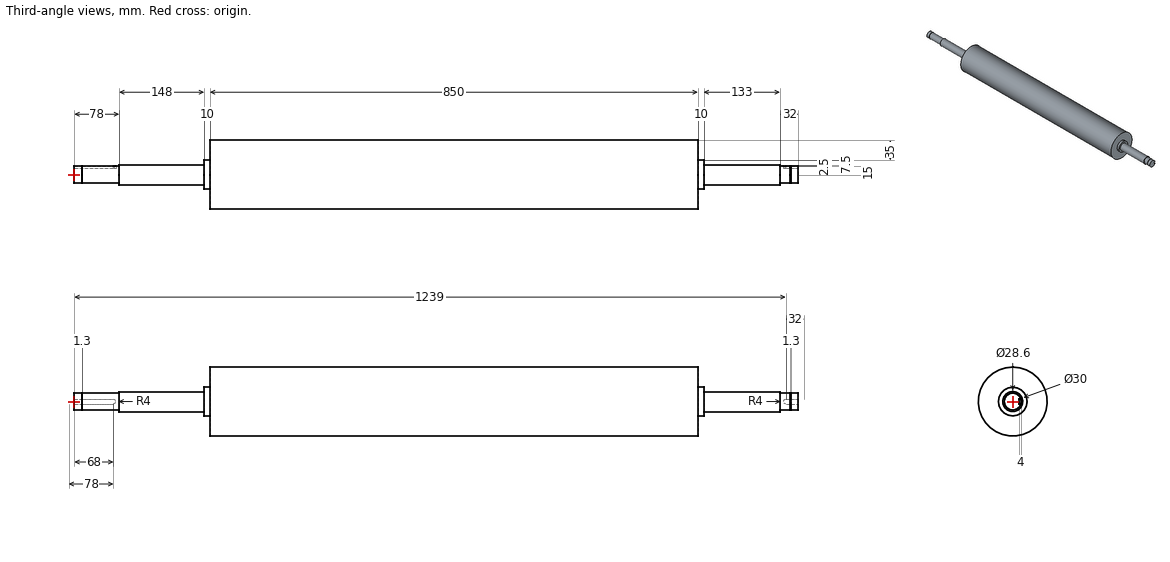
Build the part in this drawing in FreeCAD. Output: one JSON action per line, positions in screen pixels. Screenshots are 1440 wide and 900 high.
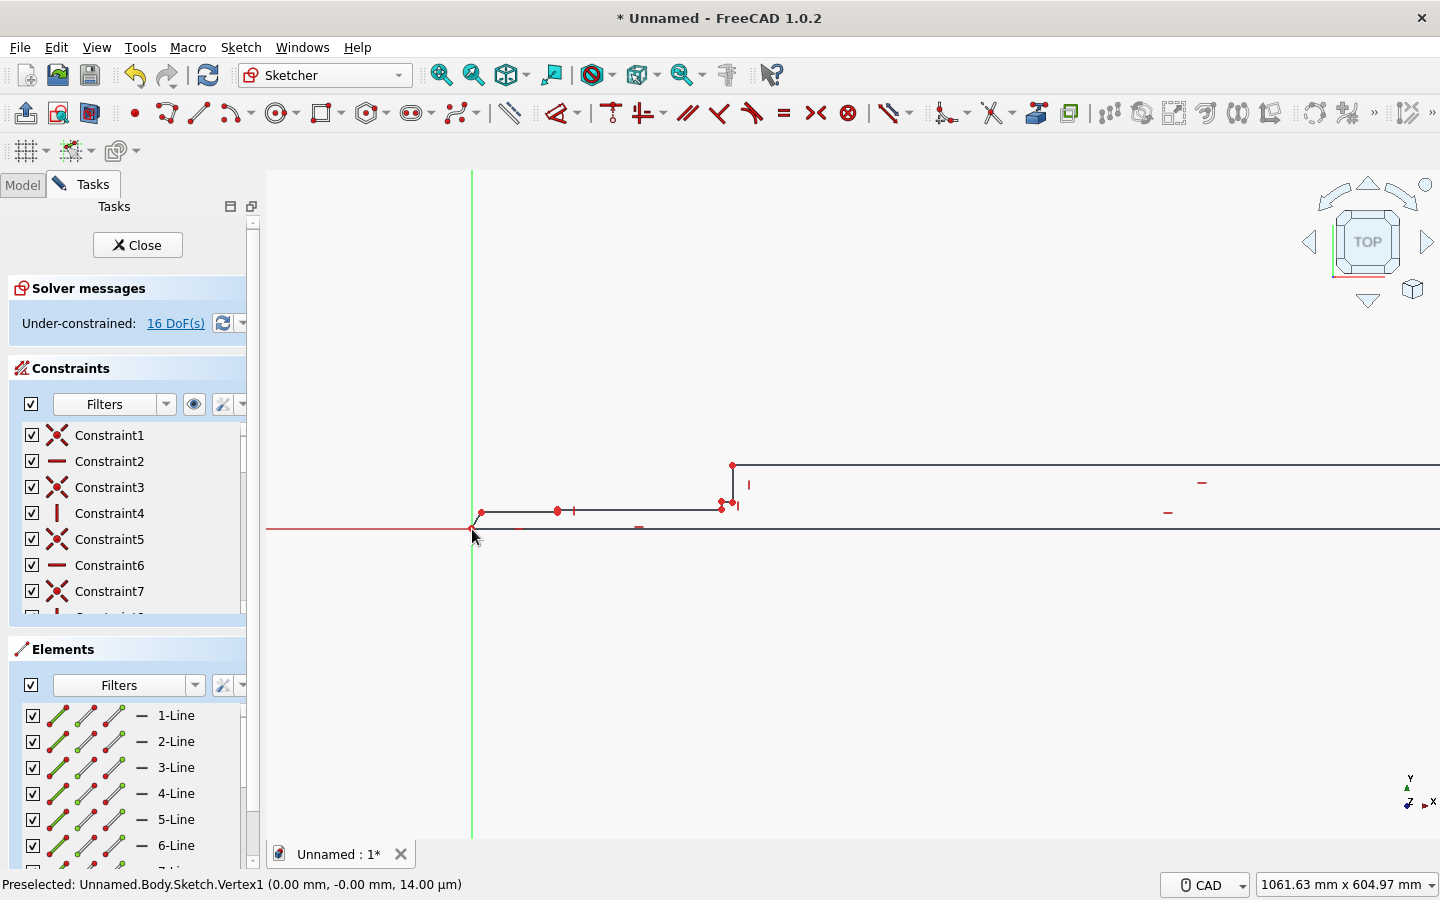
{"action": "scroll", "coordinate": [727, 502], "scroll_direction": "up", "scroll_amount": 5}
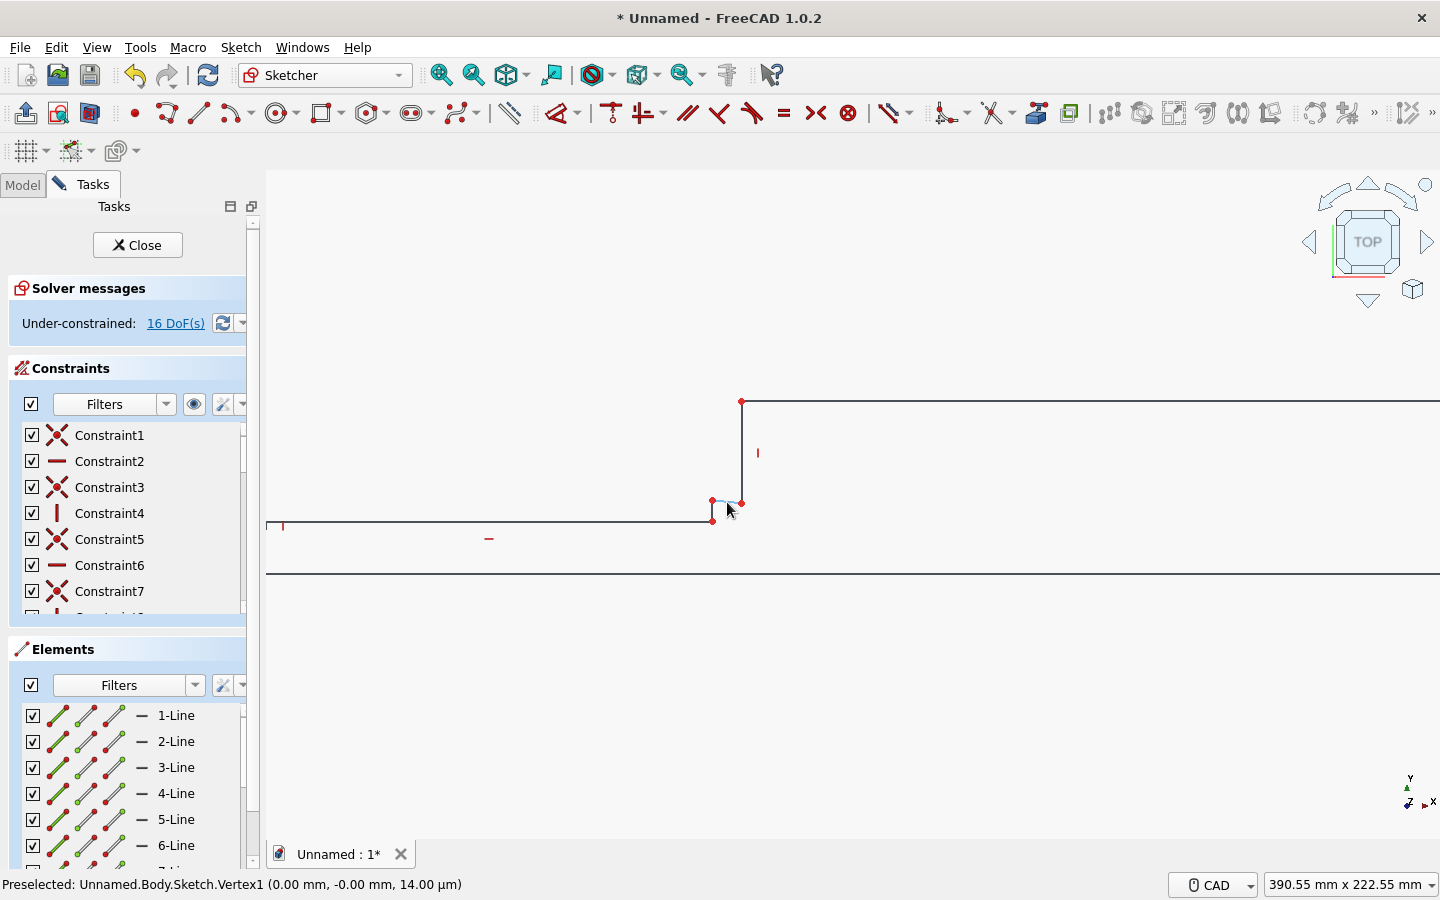
{"action": "left_click", "coordinate": [727, 502]}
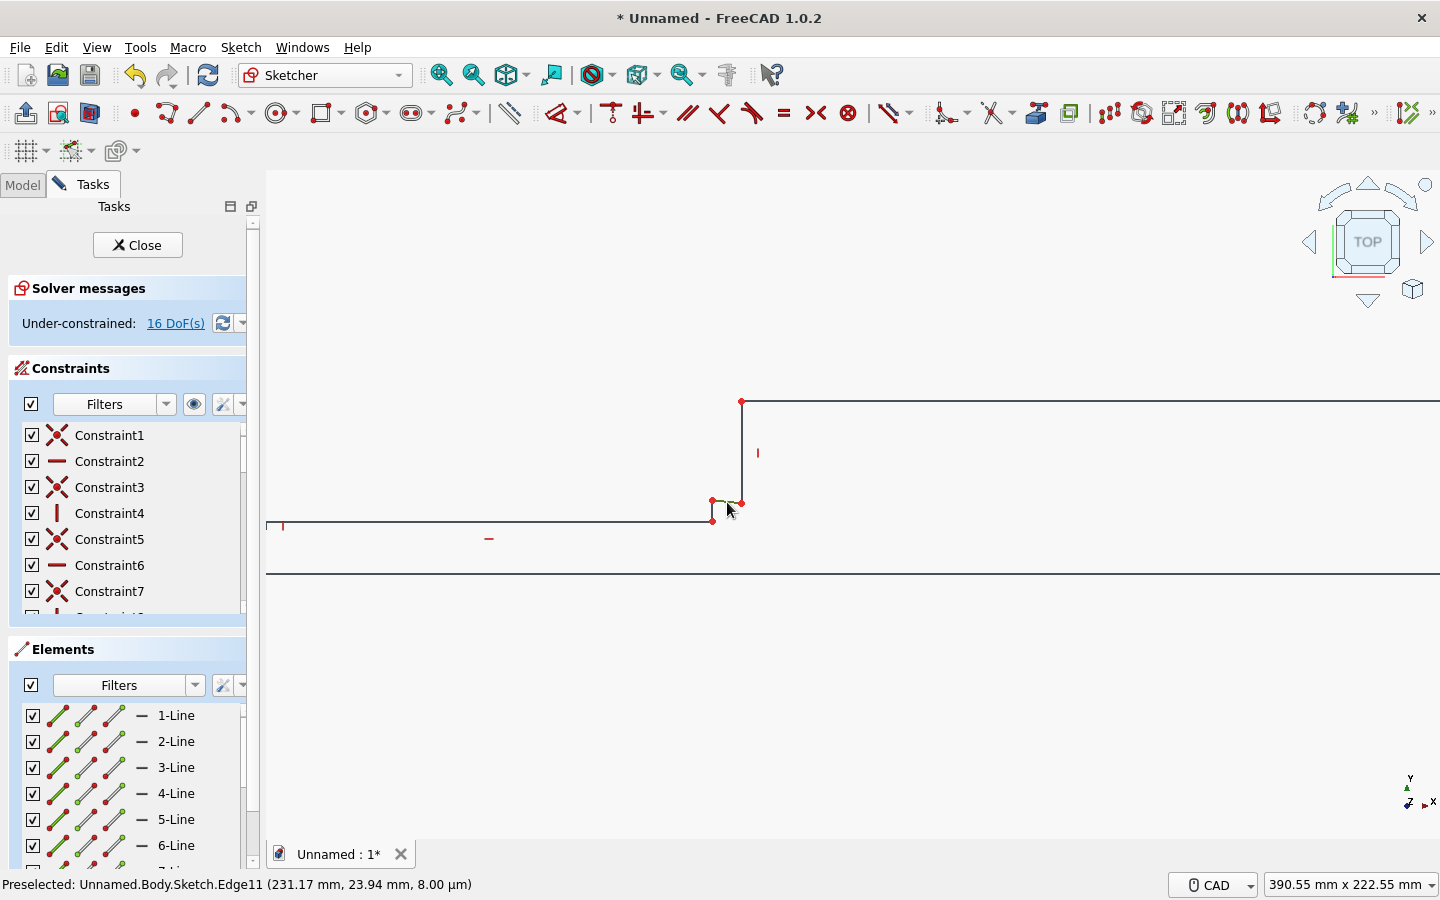
{"action": "left_click", "coordinate": [666, 114]}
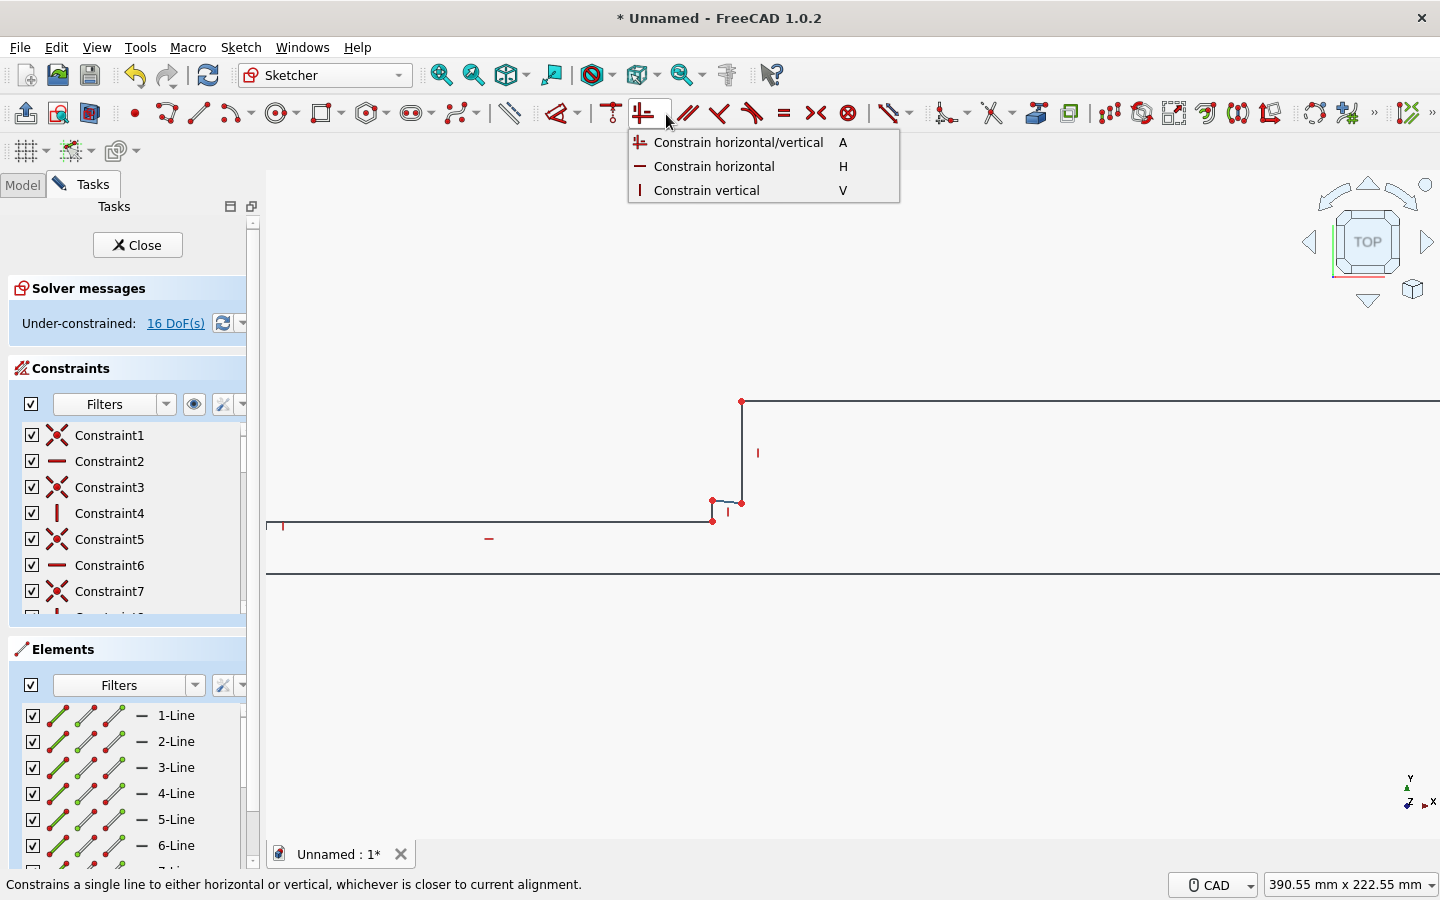
{"action": "left_click", "coordinate": [764, 166]}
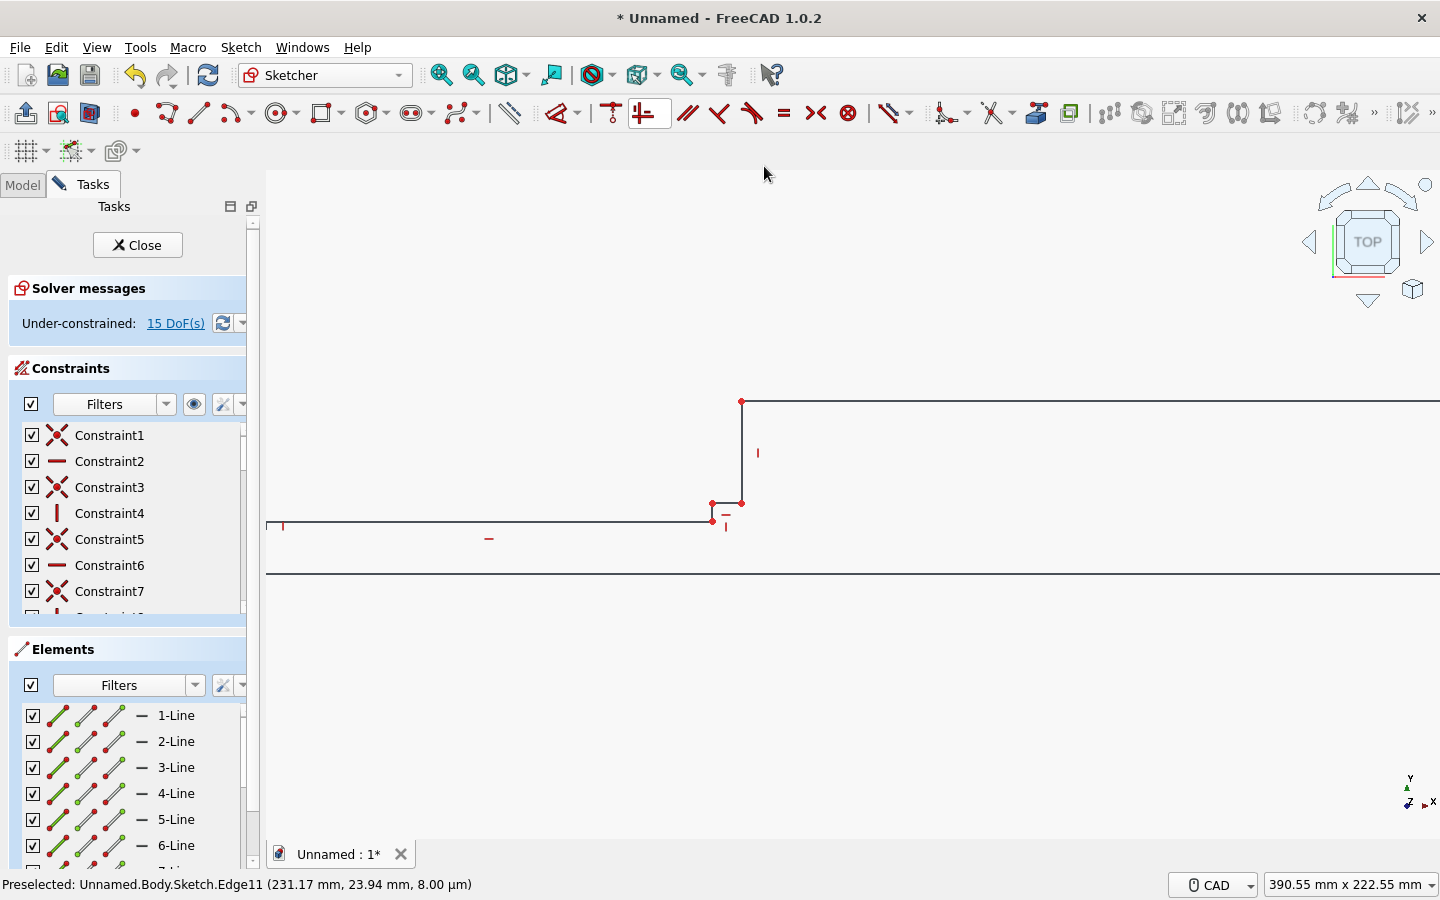
{"action": "scroll", "coordinate": [558, 509], "scroll_direction": "down", "scroll_amount": 9}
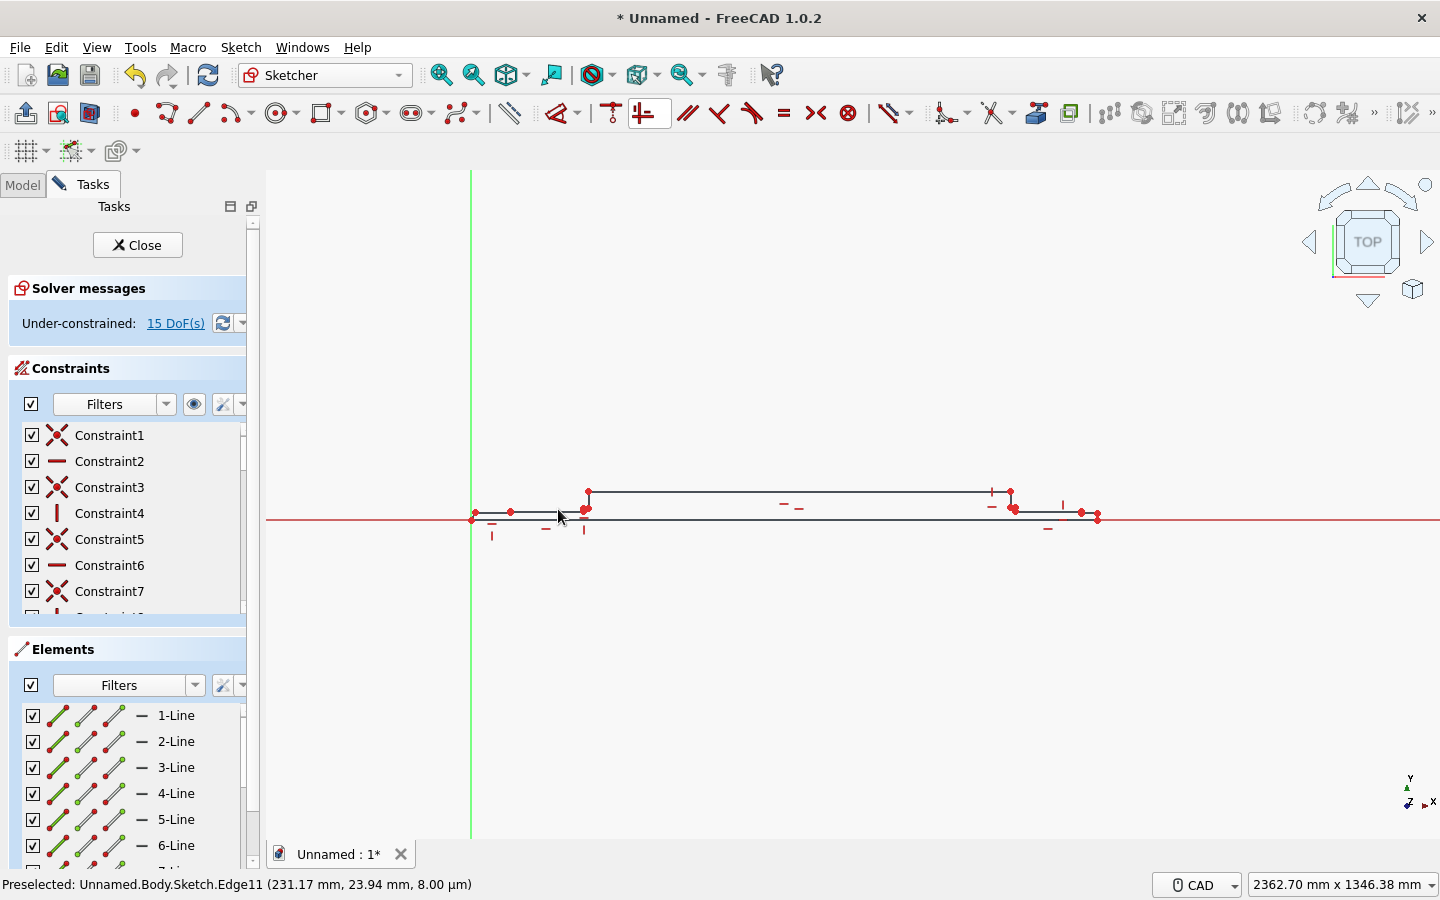
{"action": "scroll", "coordinate": [474, 515], "scroll_direction": "up", "scroll_amount": 9}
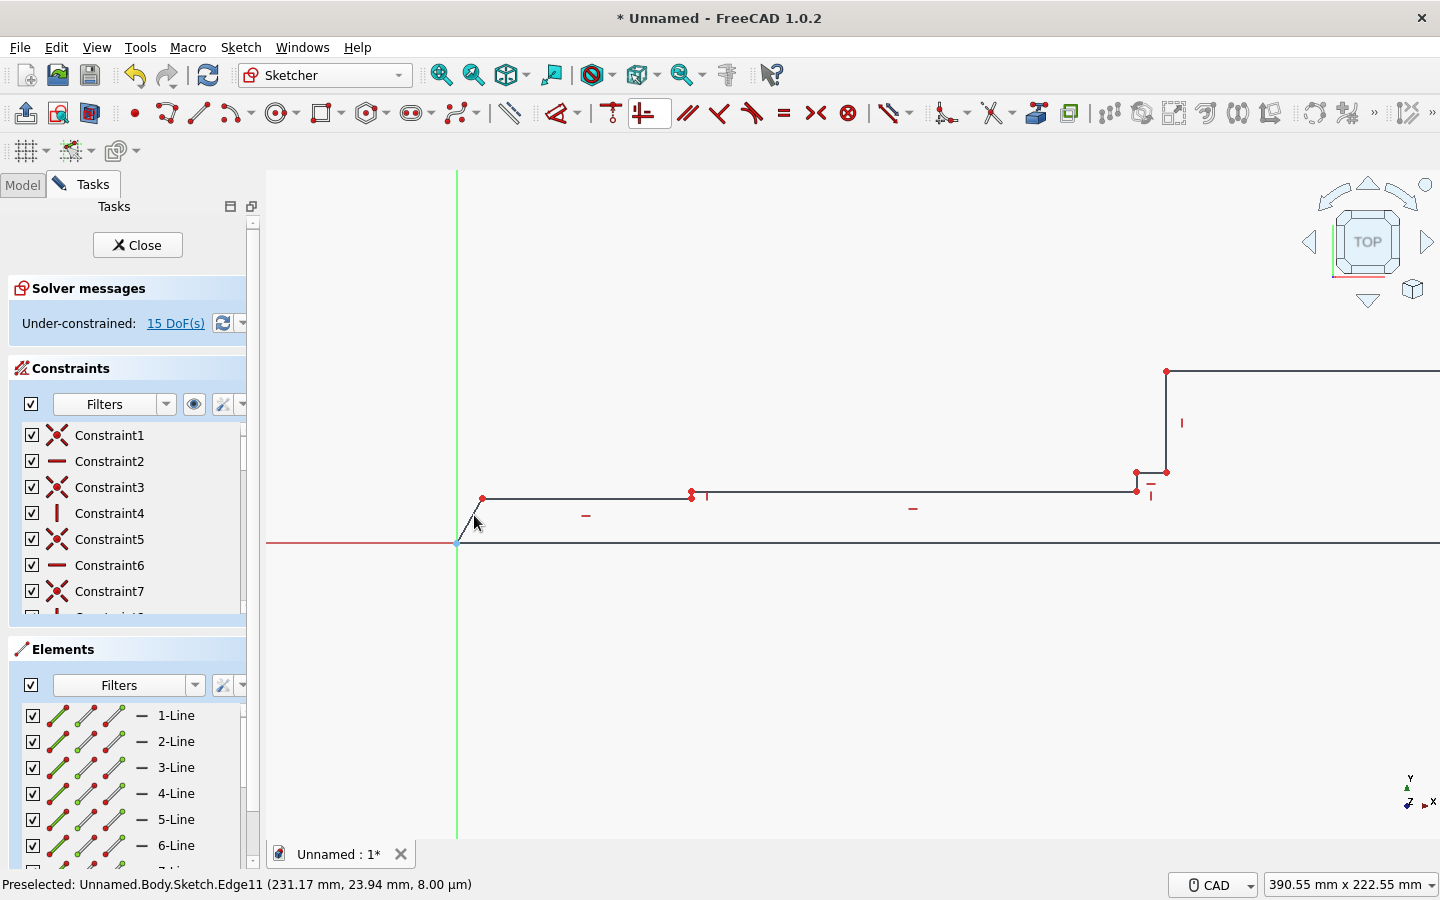
{"action": "left_click", "coordinate": [475, 512]}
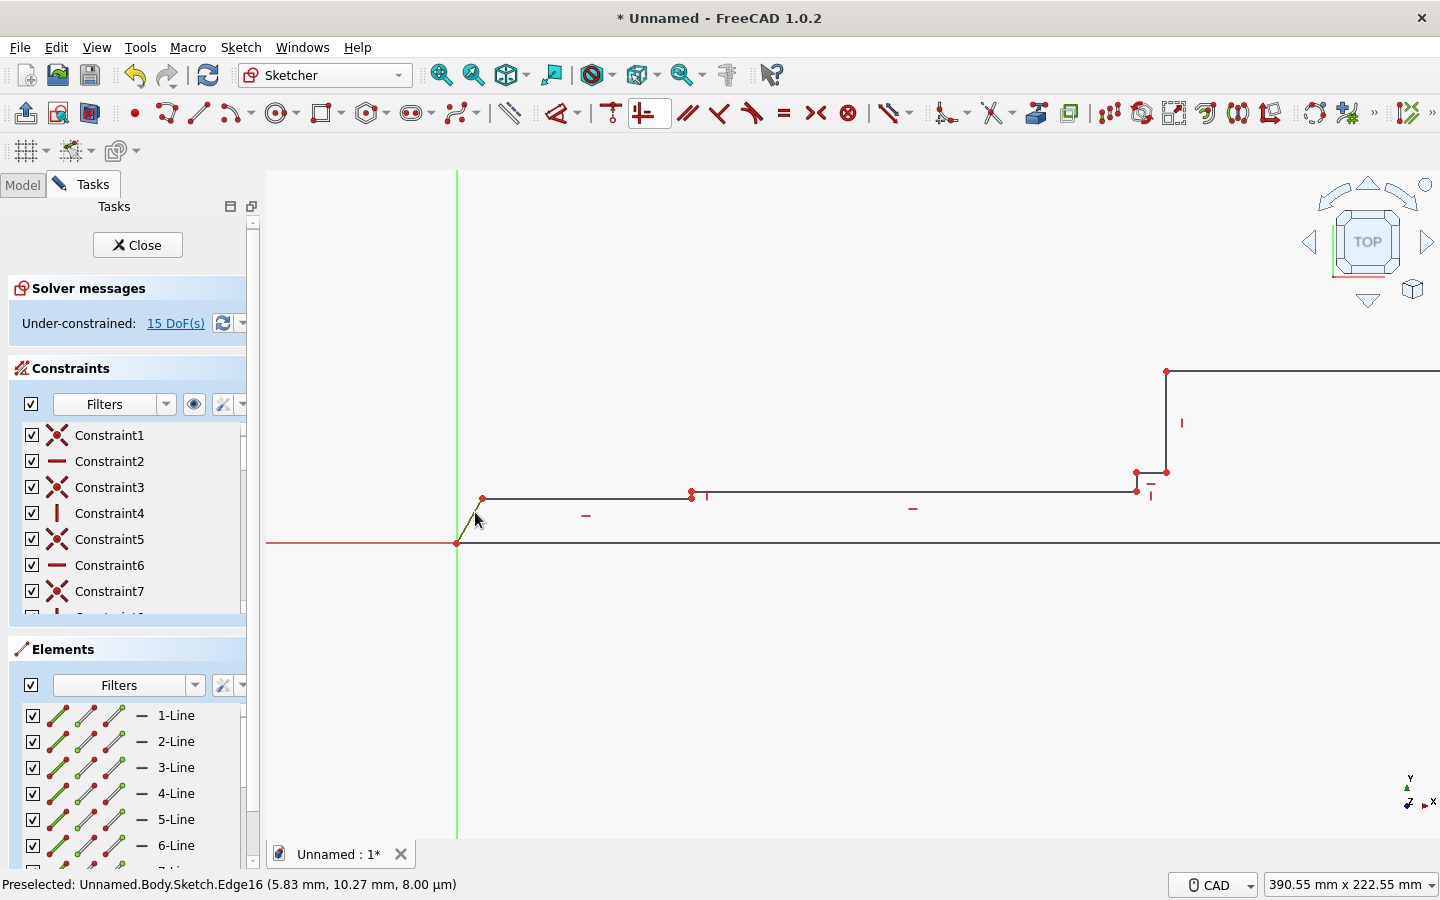
{"action": "key", "text": "v"}